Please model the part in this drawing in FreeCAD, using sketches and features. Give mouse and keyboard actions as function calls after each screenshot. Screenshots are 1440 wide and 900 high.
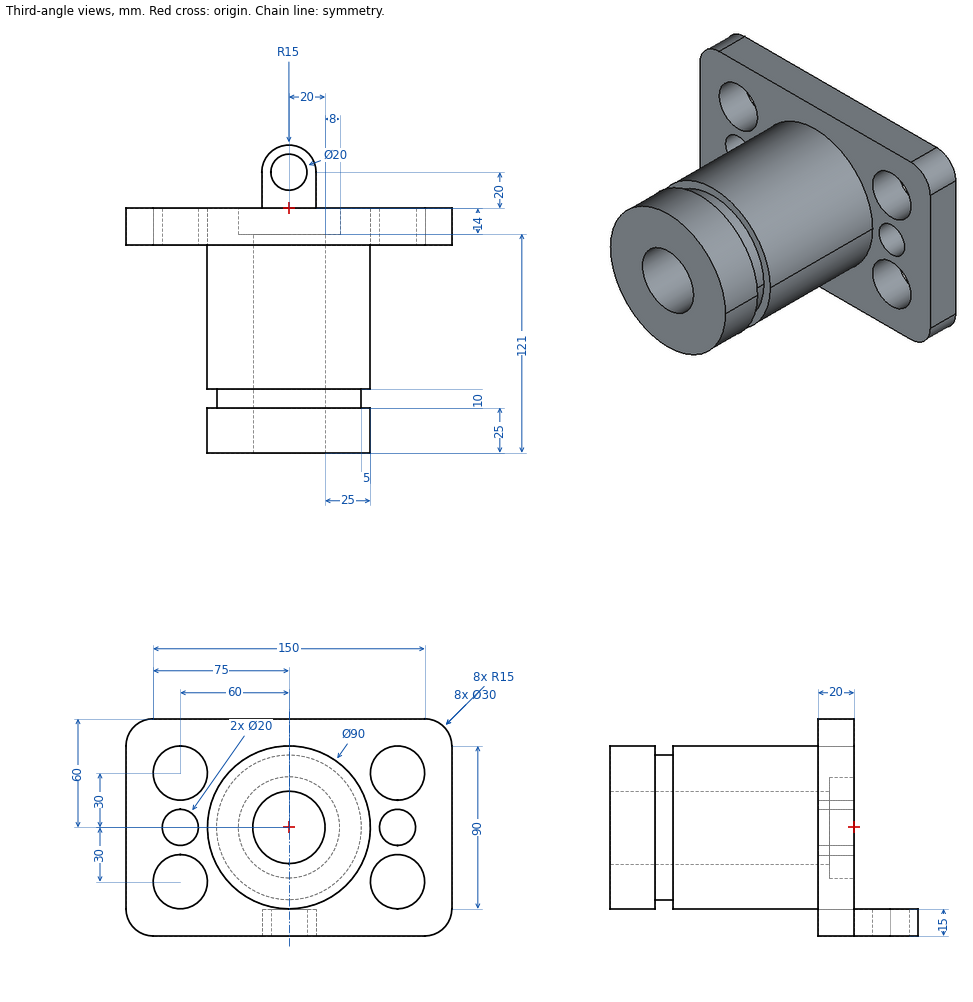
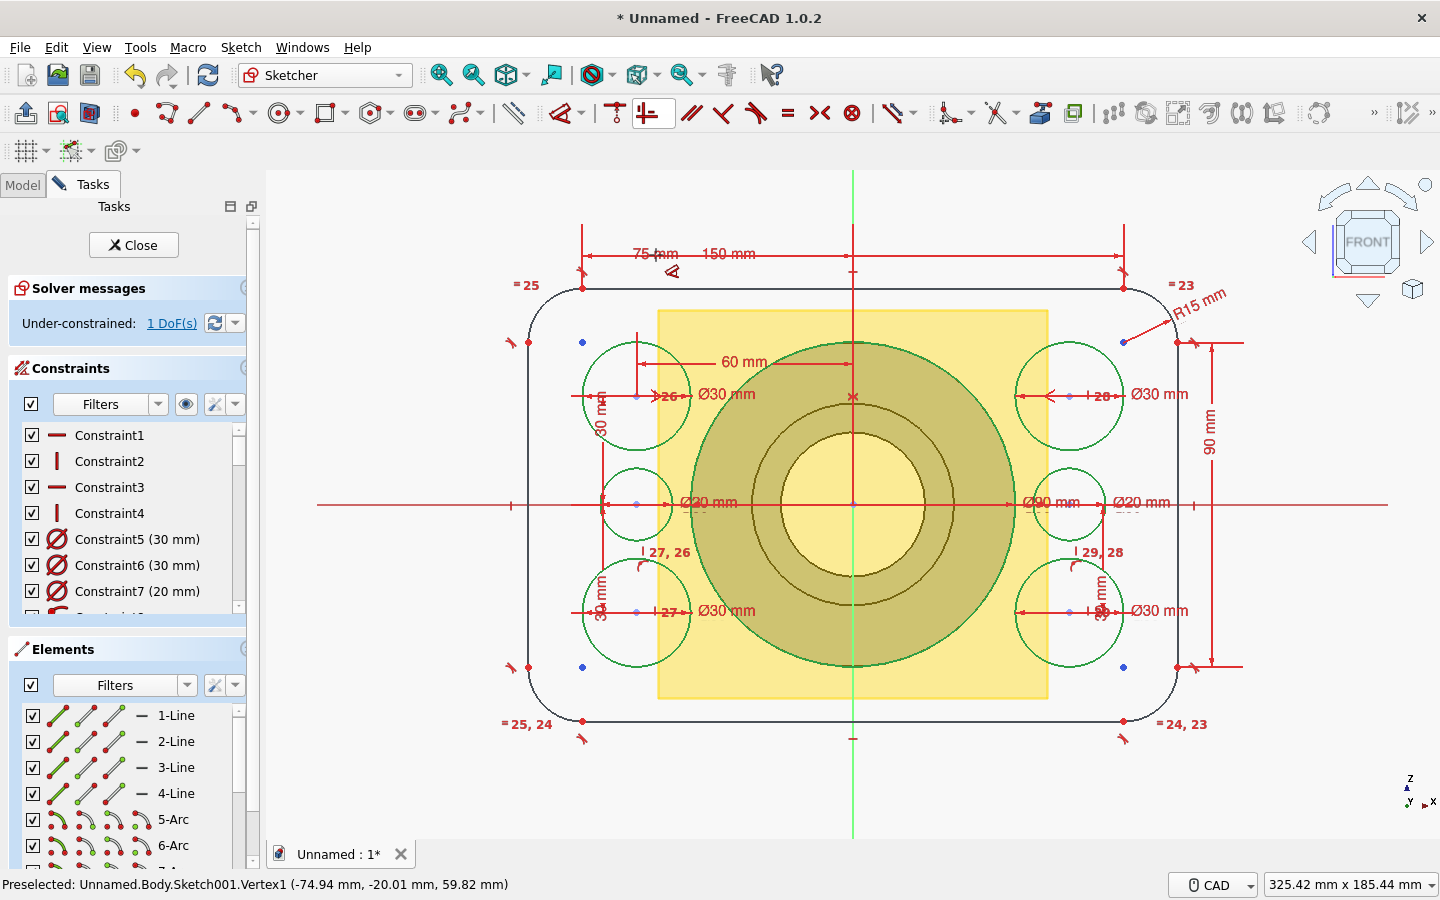
click(582, 289)
click(548, 347)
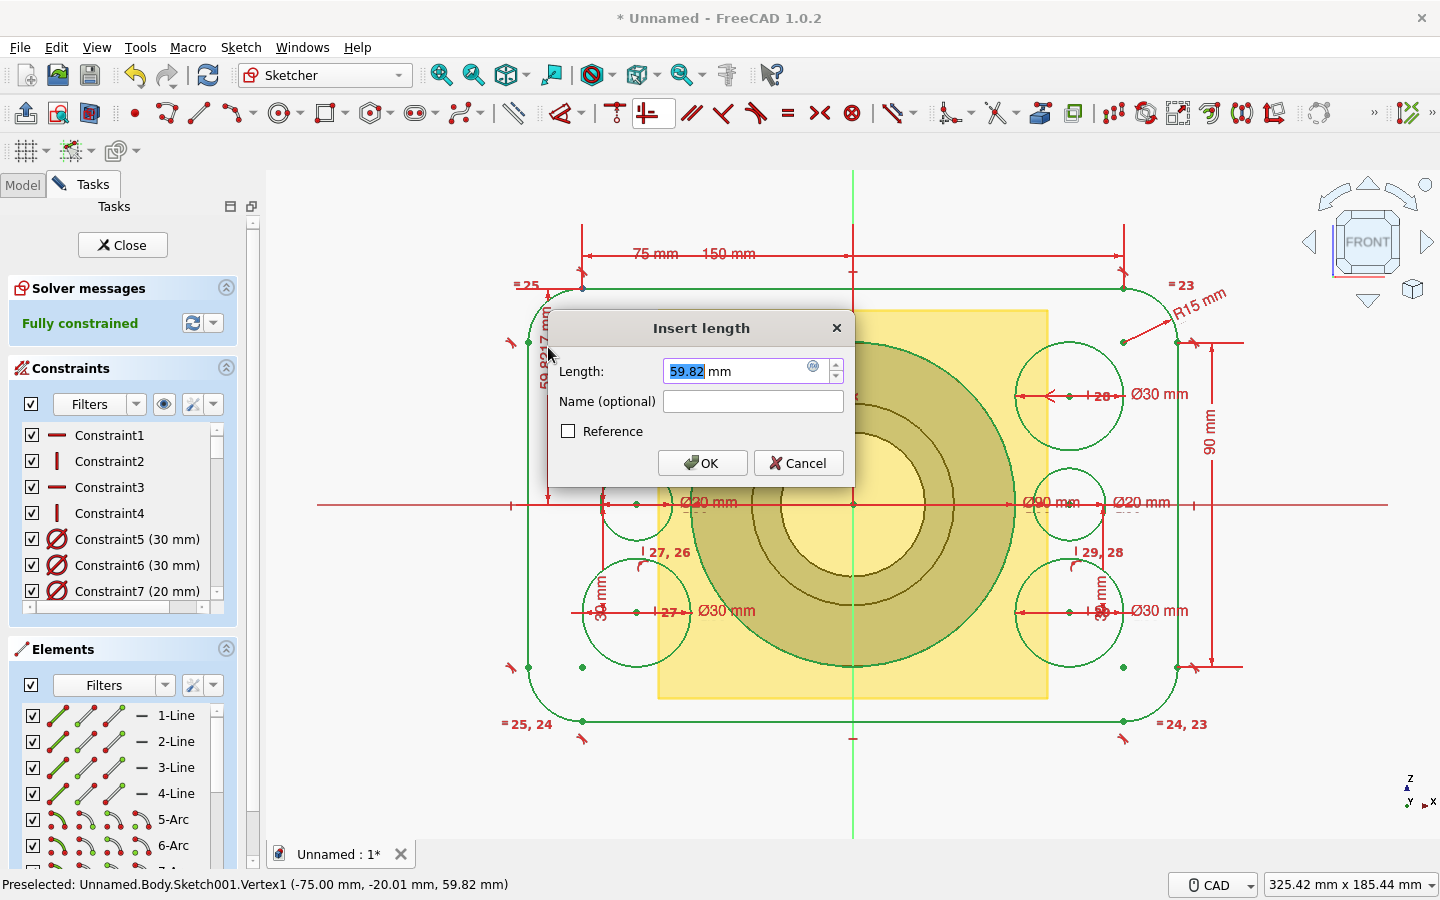
text(60)
key(Return)
key(Escape)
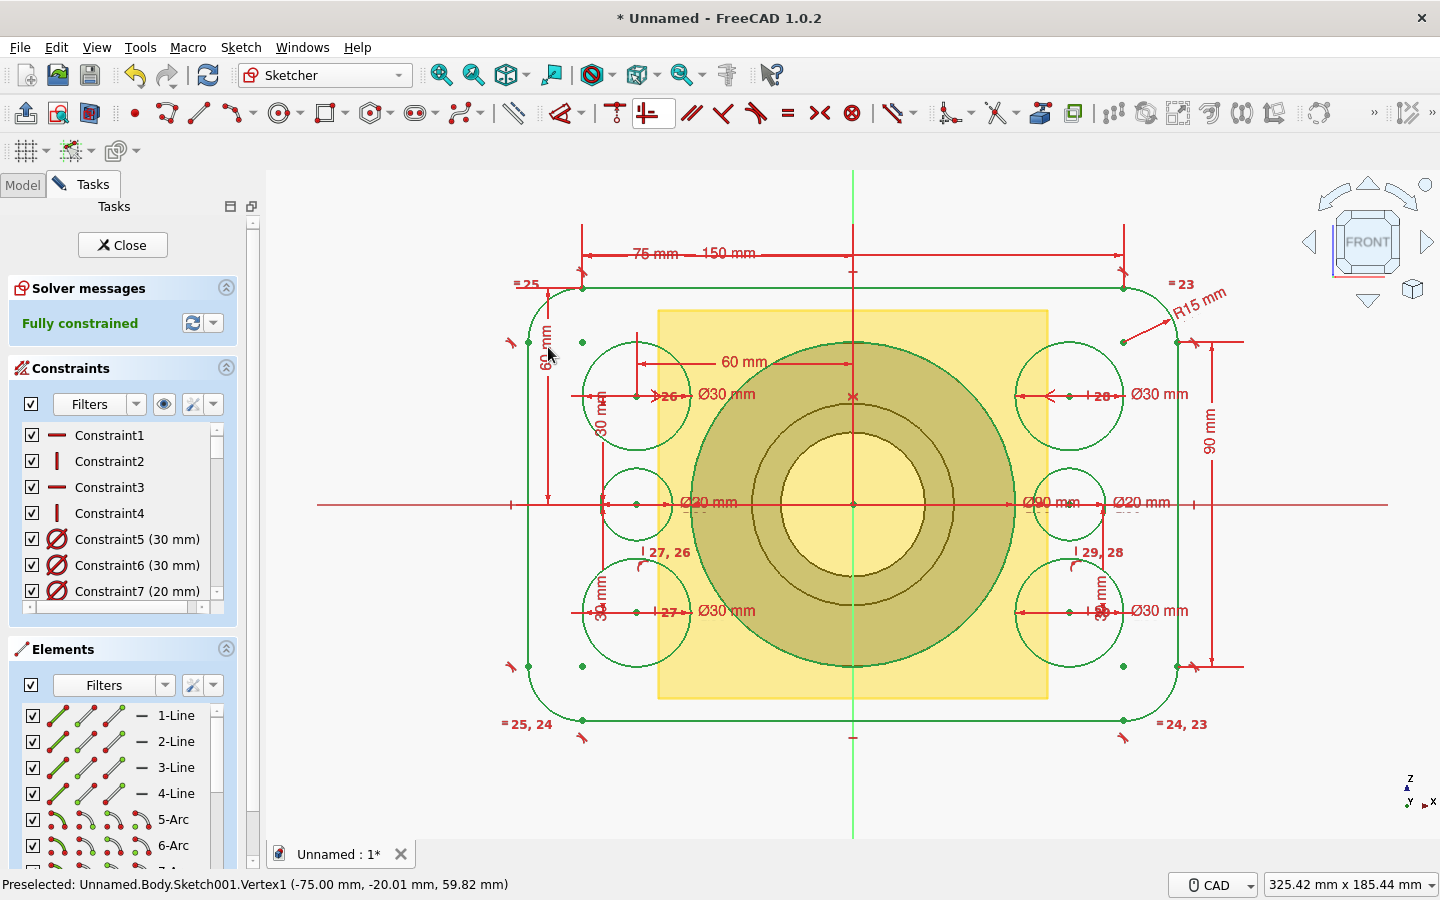
click(123, 245)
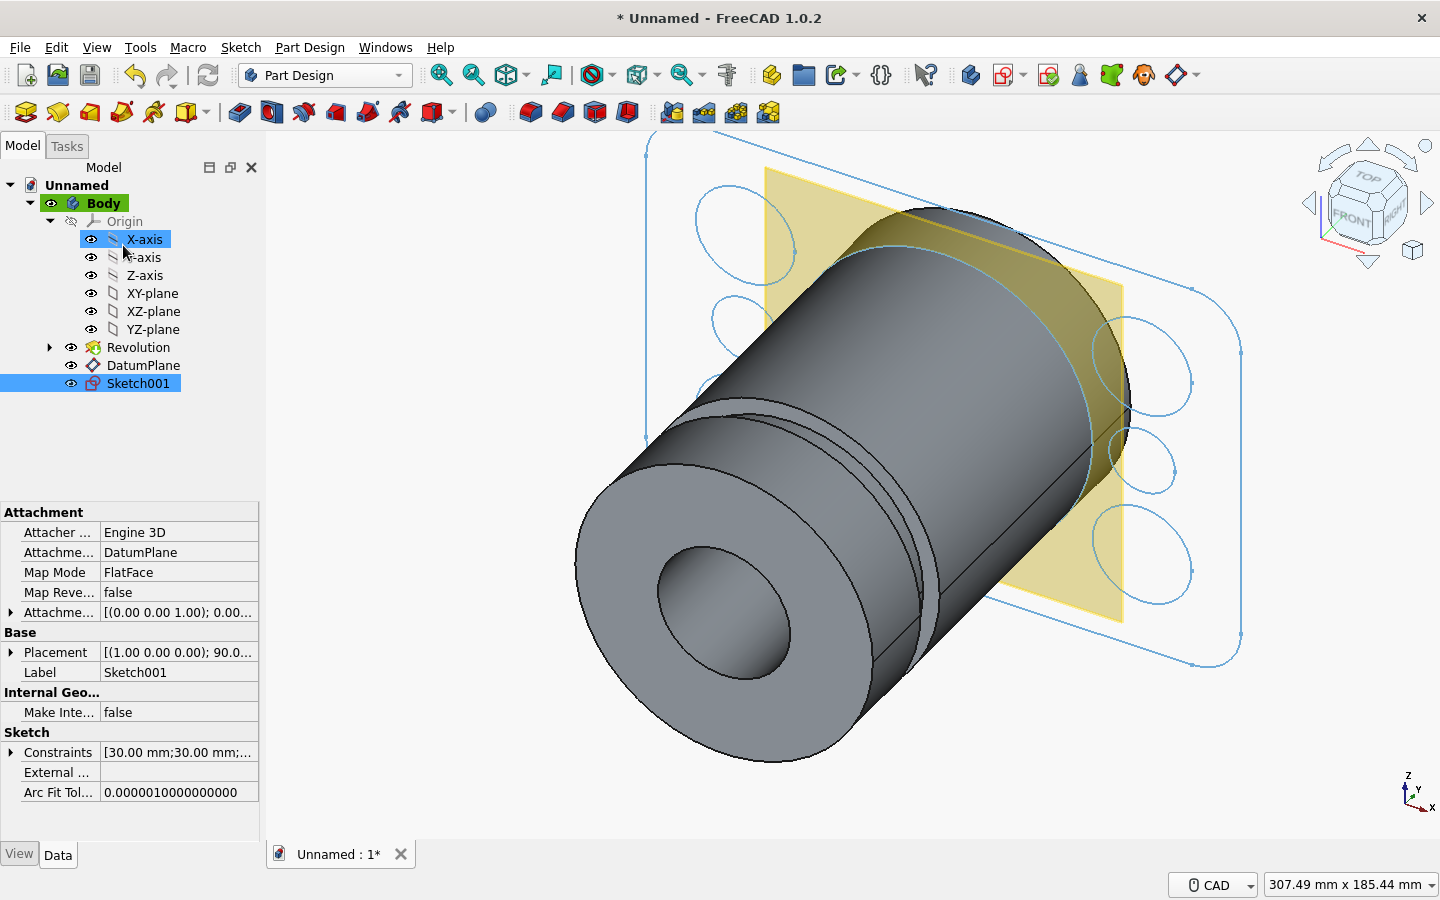
click(26, 112)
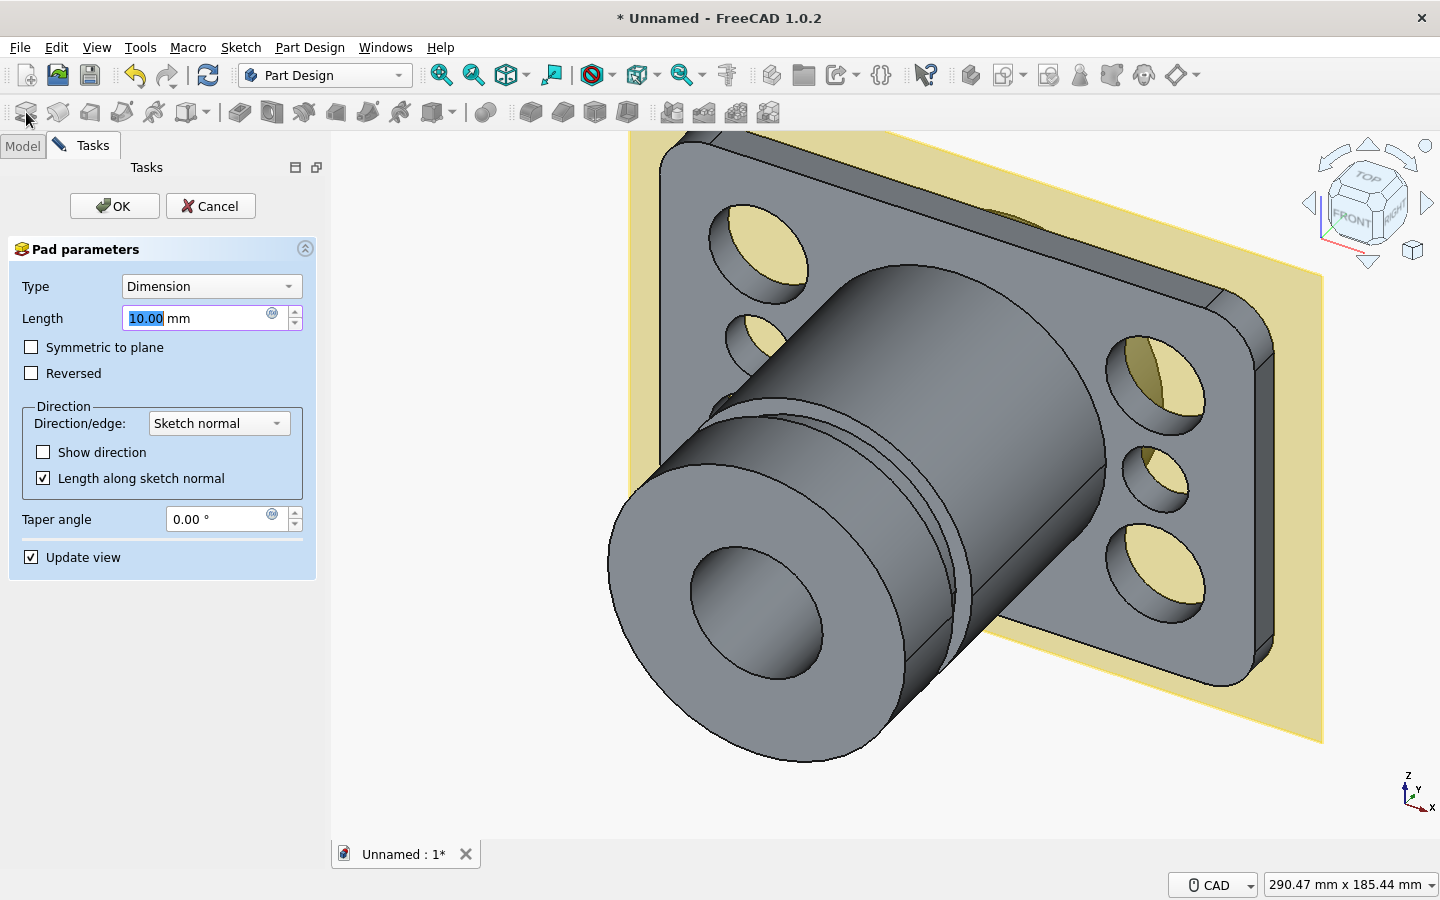
text(20)
key(Tab)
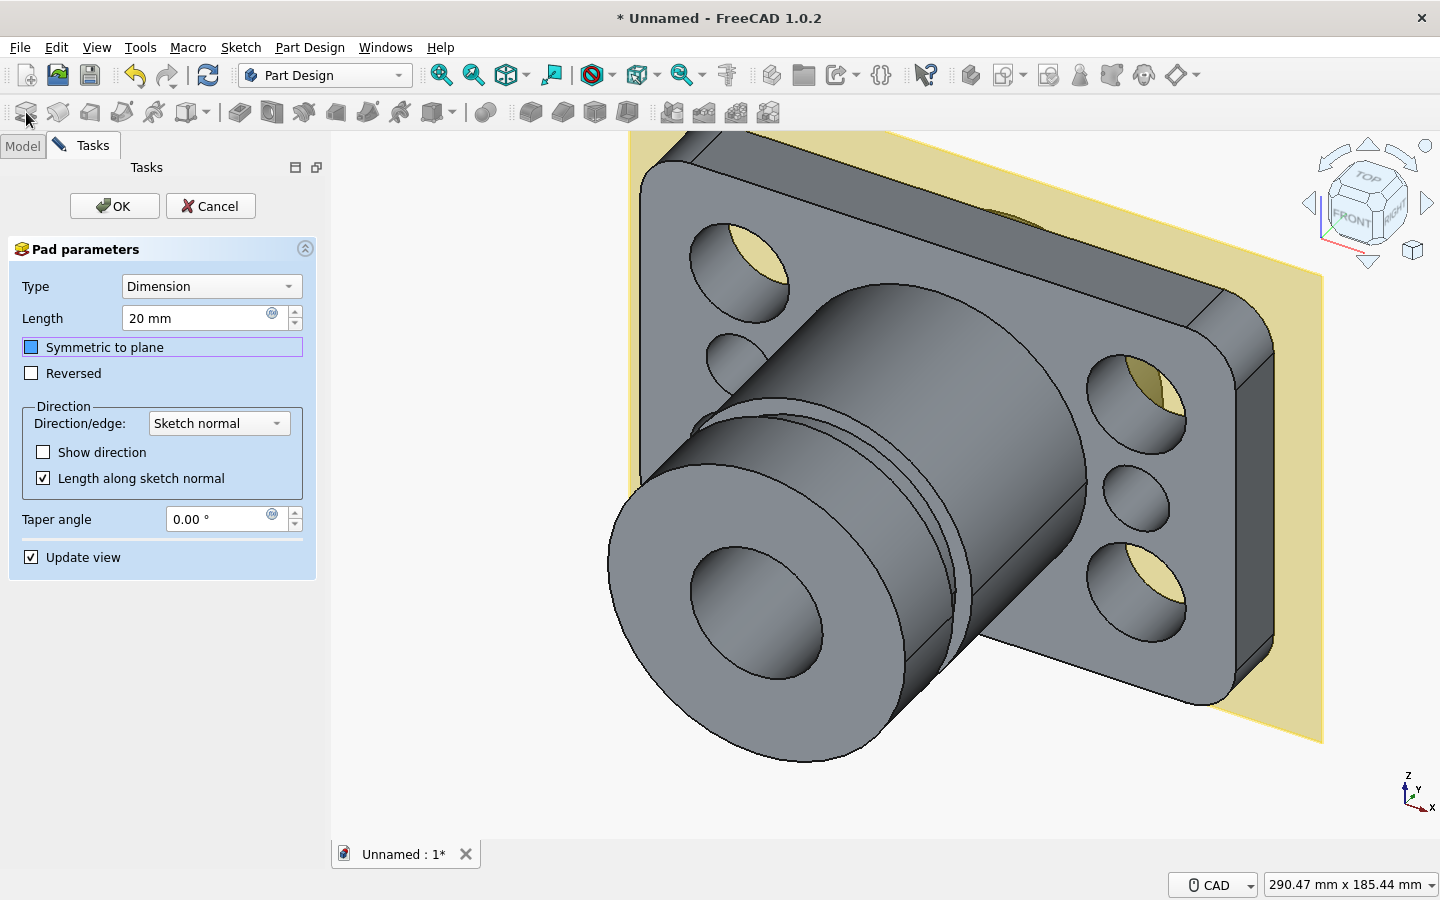
click(30, 373)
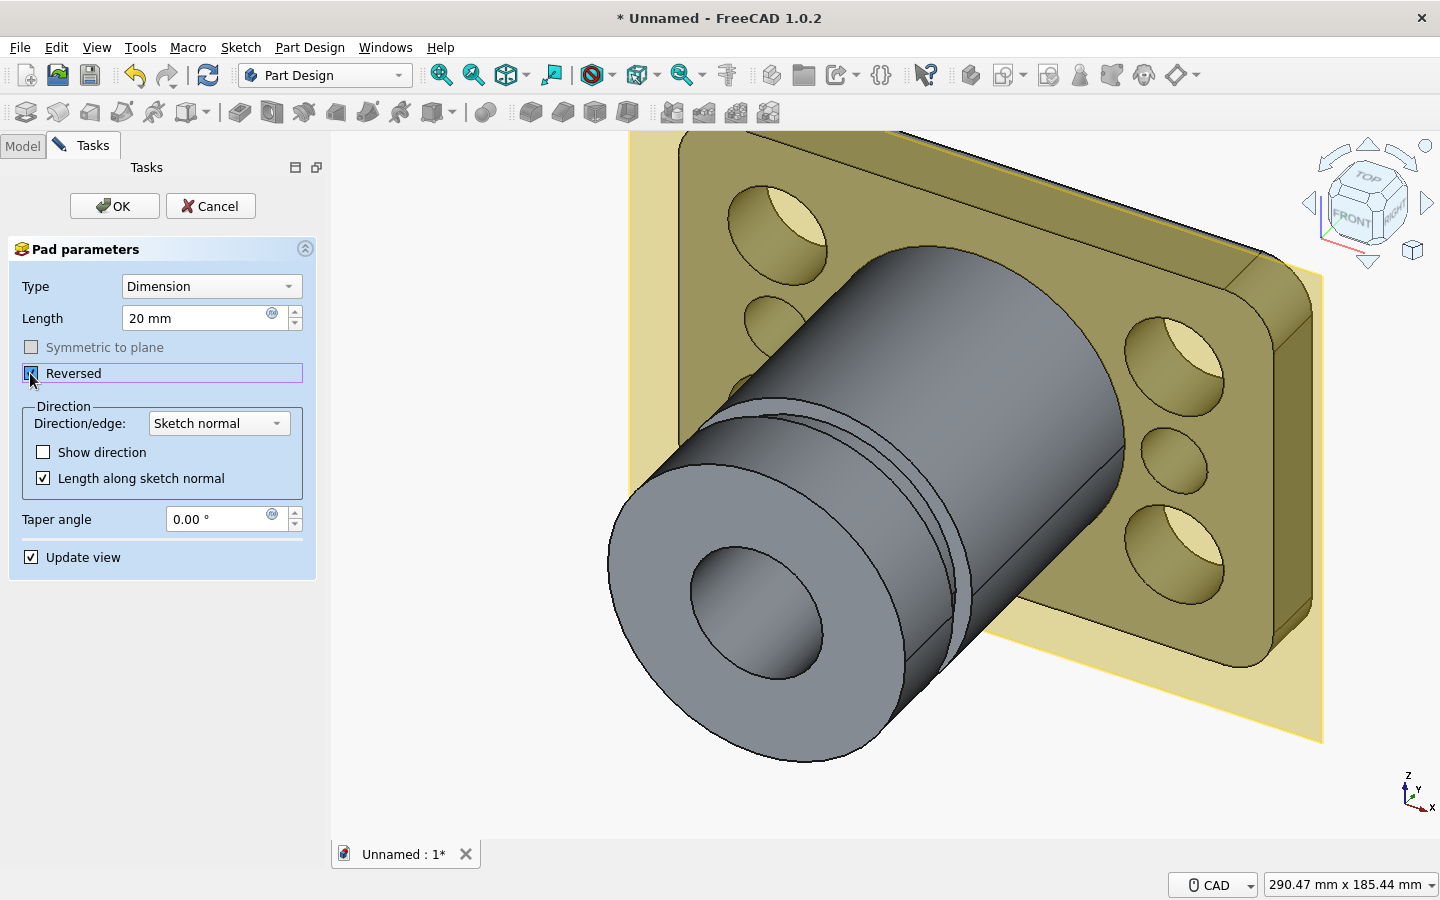
click(115, 206)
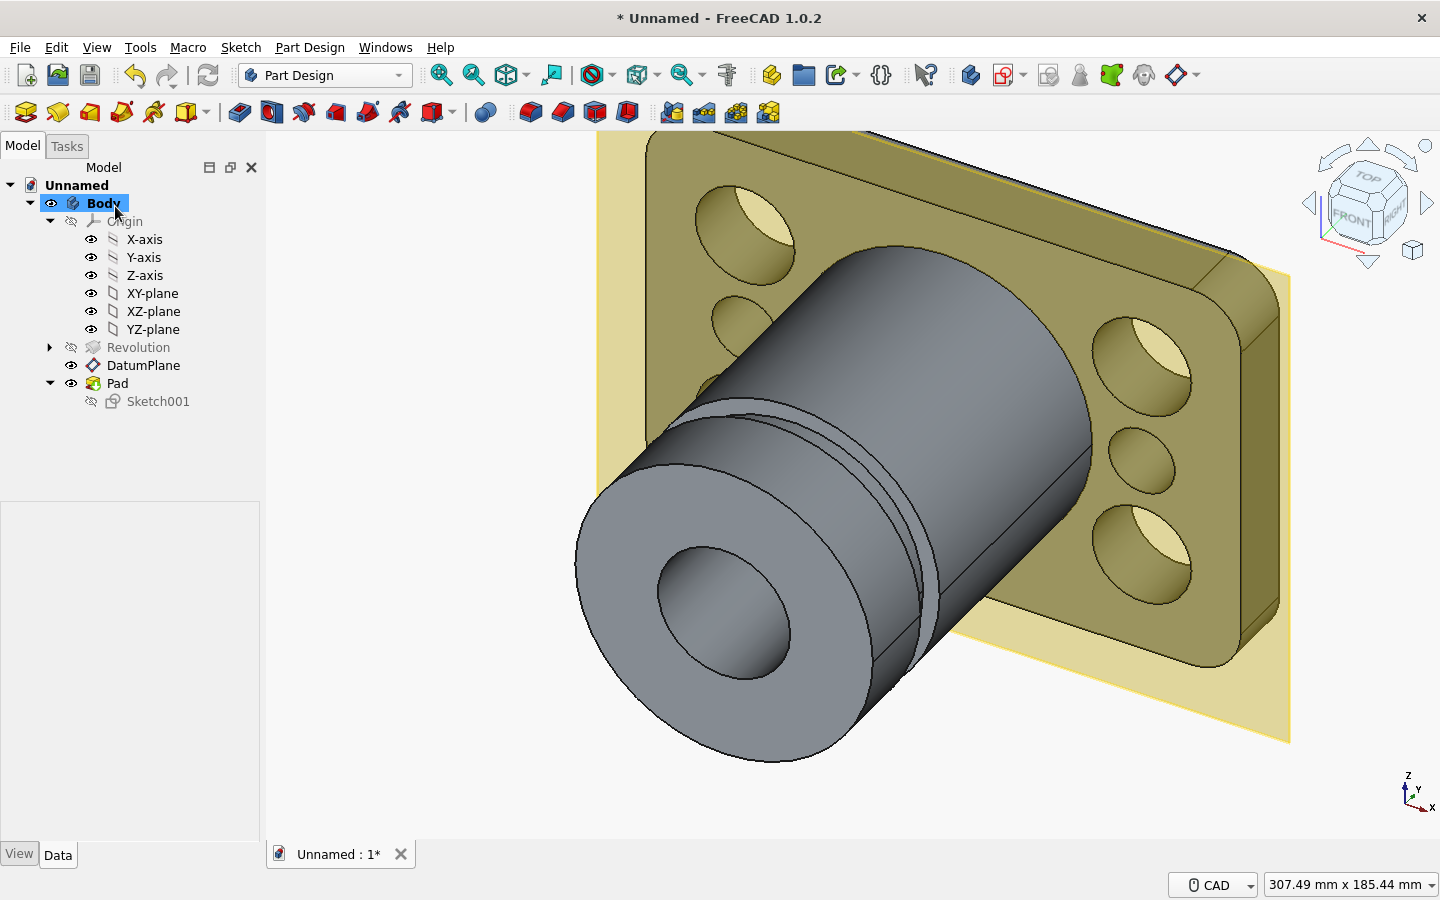
click(116, 365)
key(space)